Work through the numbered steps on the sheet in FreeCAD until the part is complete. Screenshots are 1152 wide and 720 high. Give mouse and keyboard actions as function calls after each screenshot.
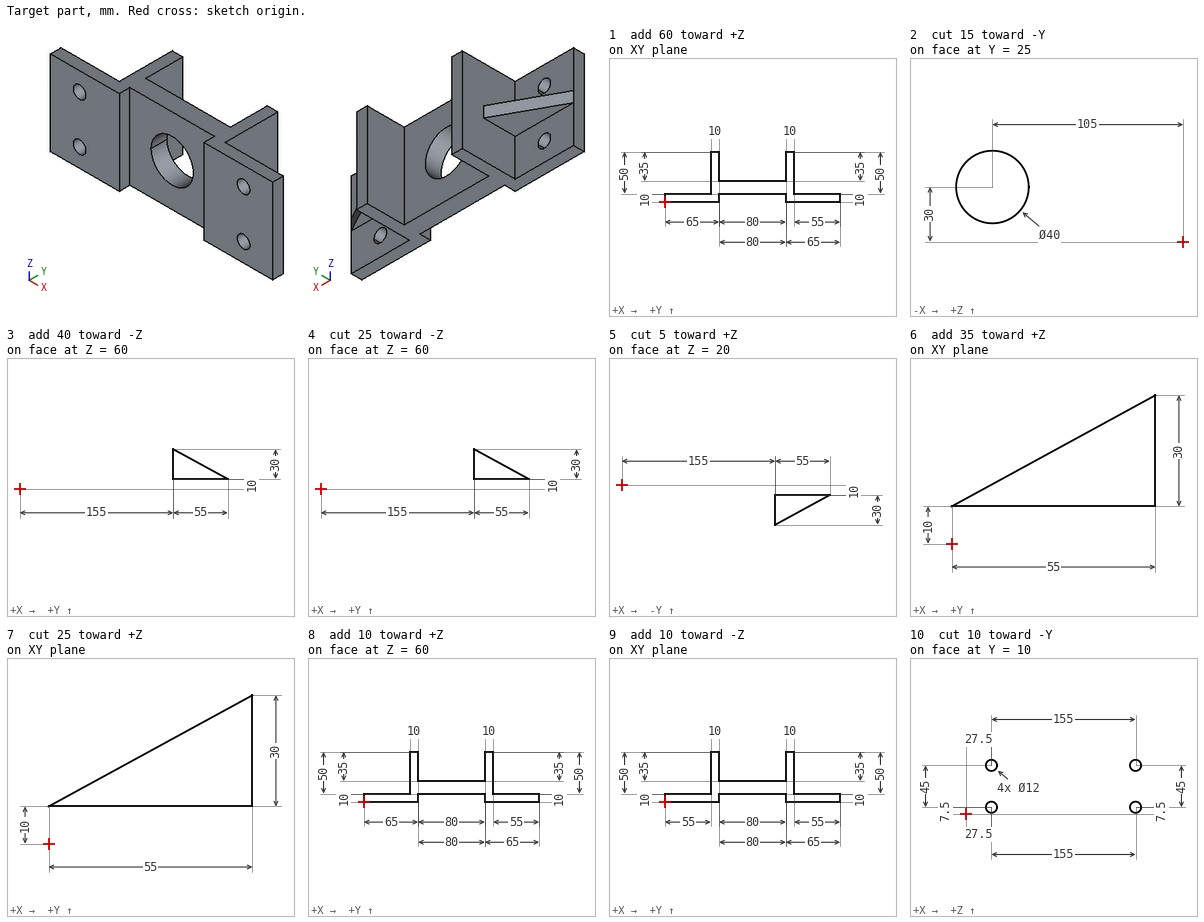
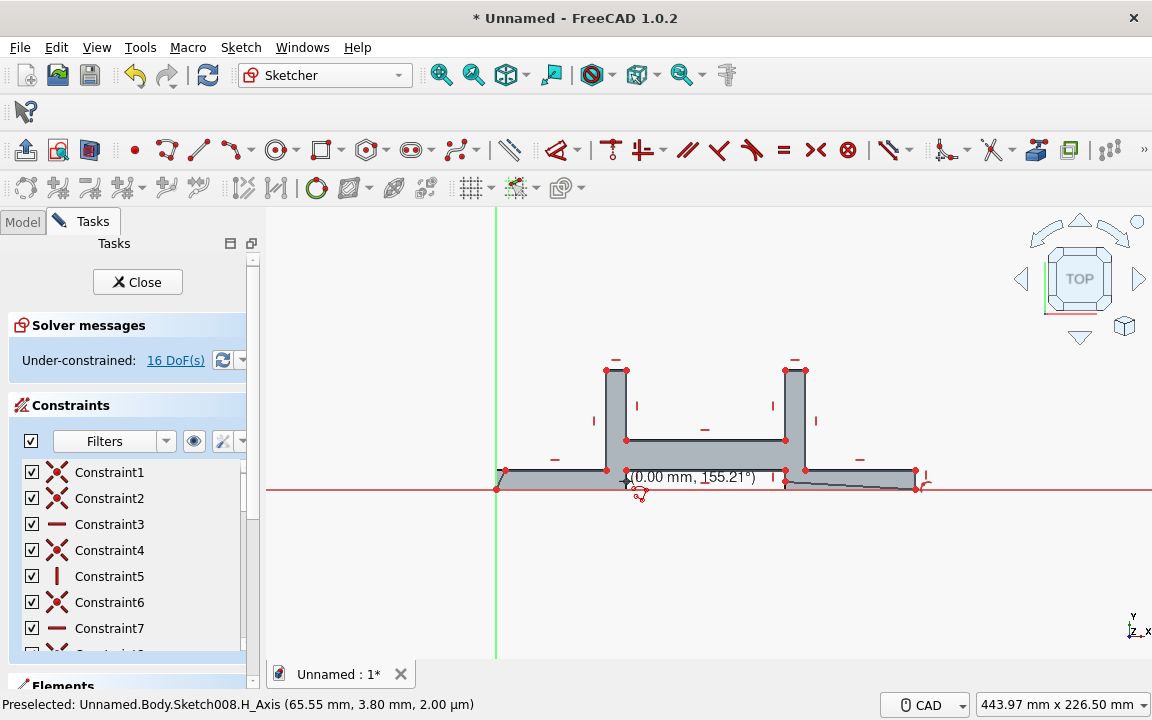
scroll(496, 490, up, 3)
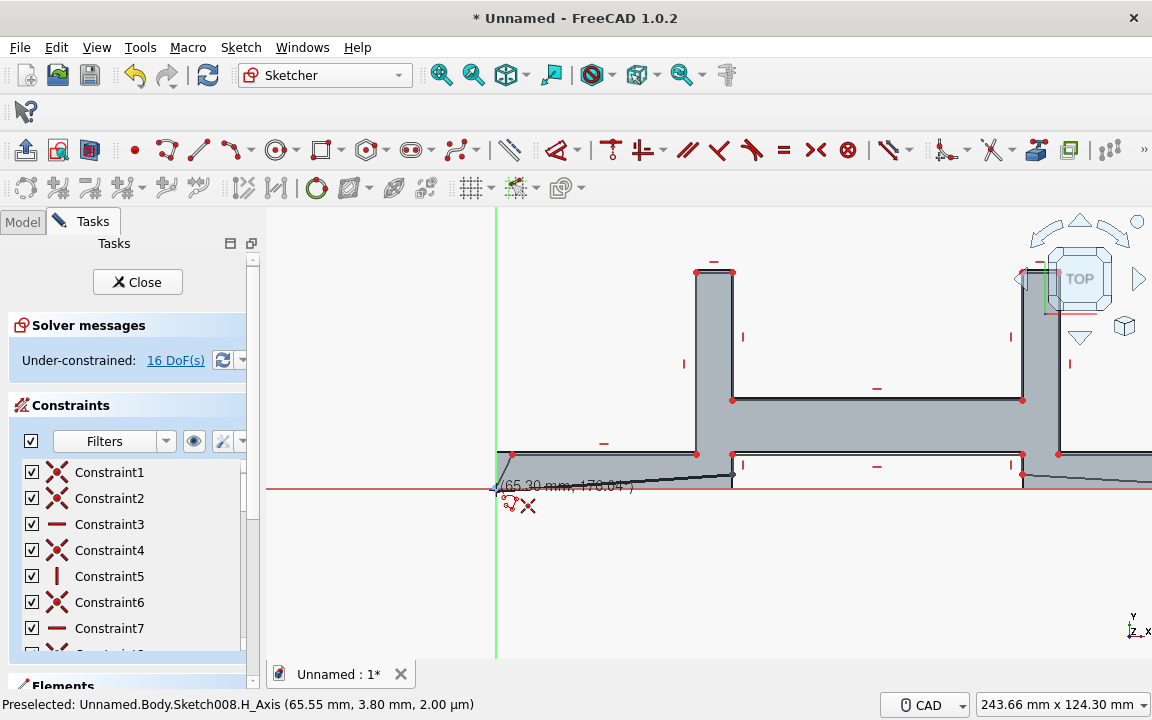
click(496, 489)
key(Escape)
key(Escape)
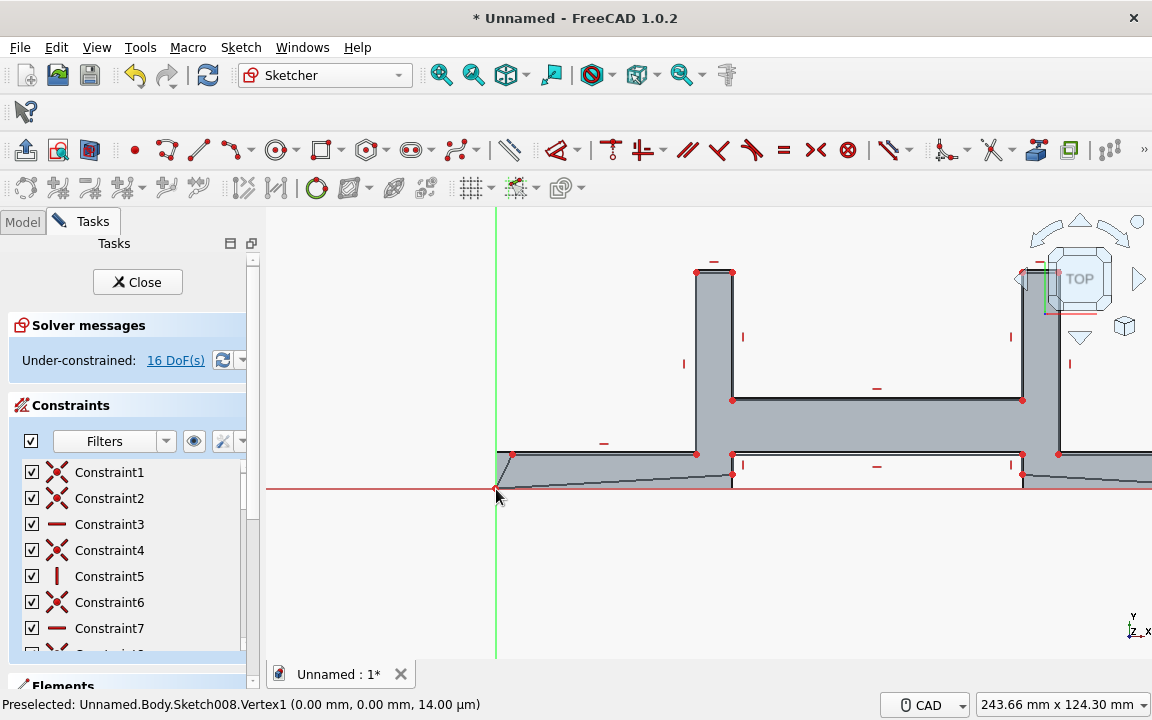
scroll(507, 465, up, 2)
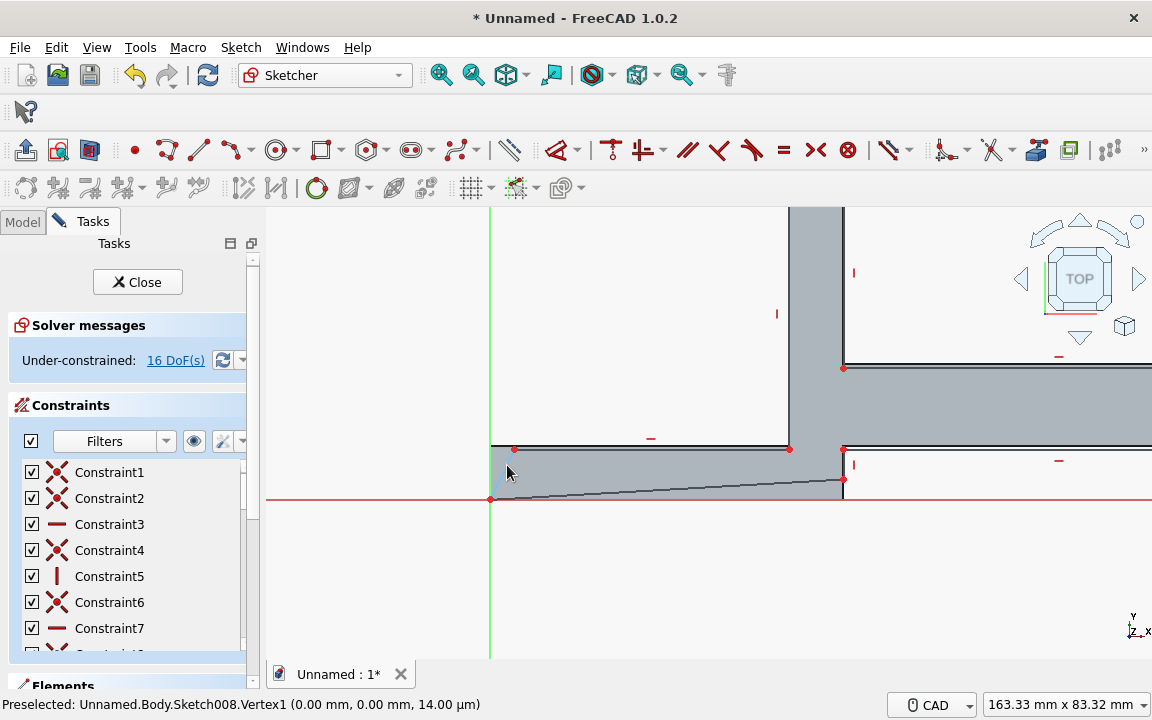
click(507, 465)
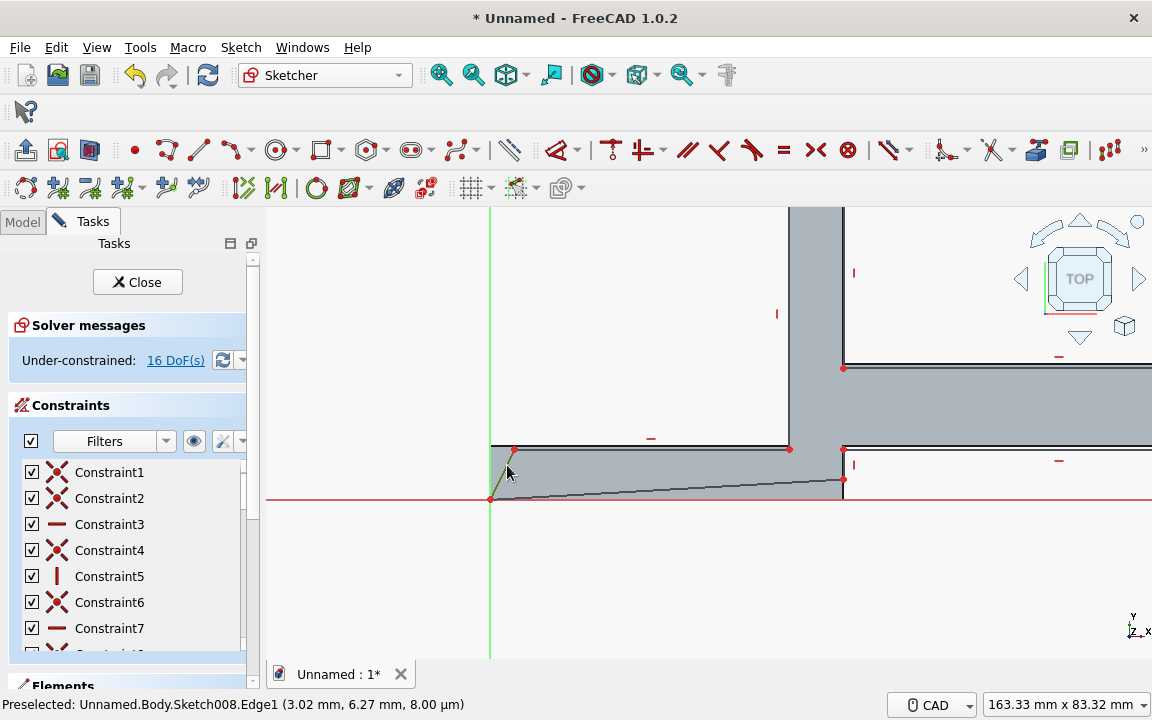
key(v)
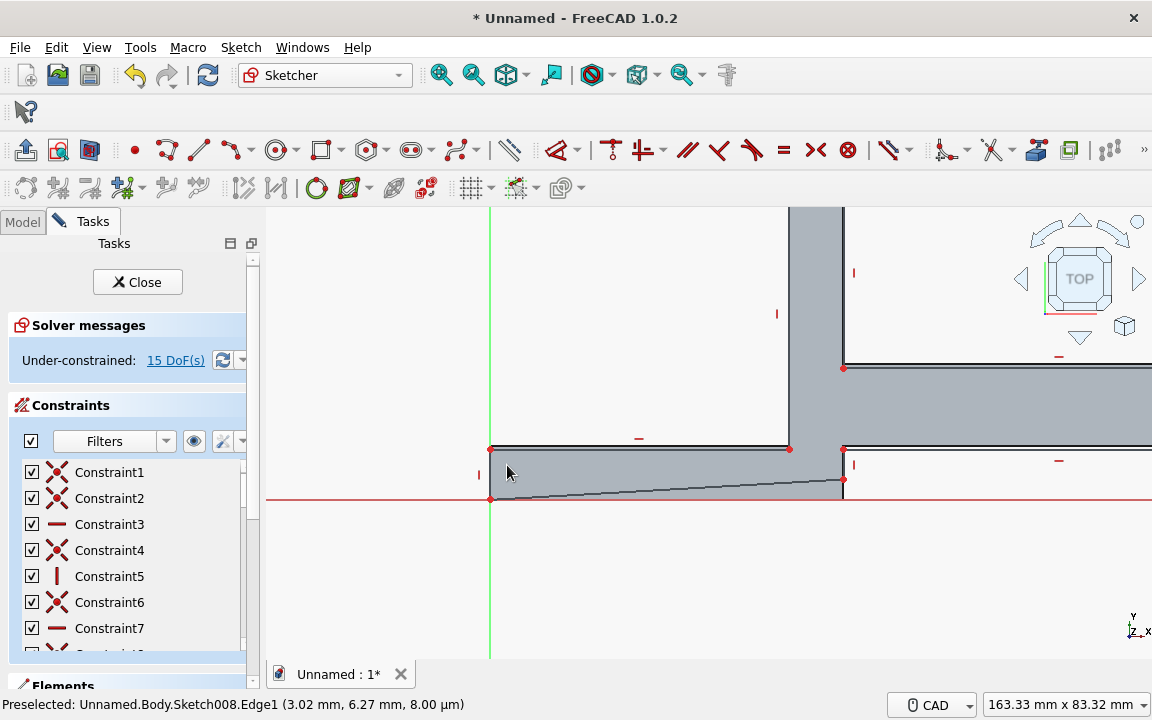
scroll(298, 511, down, 4)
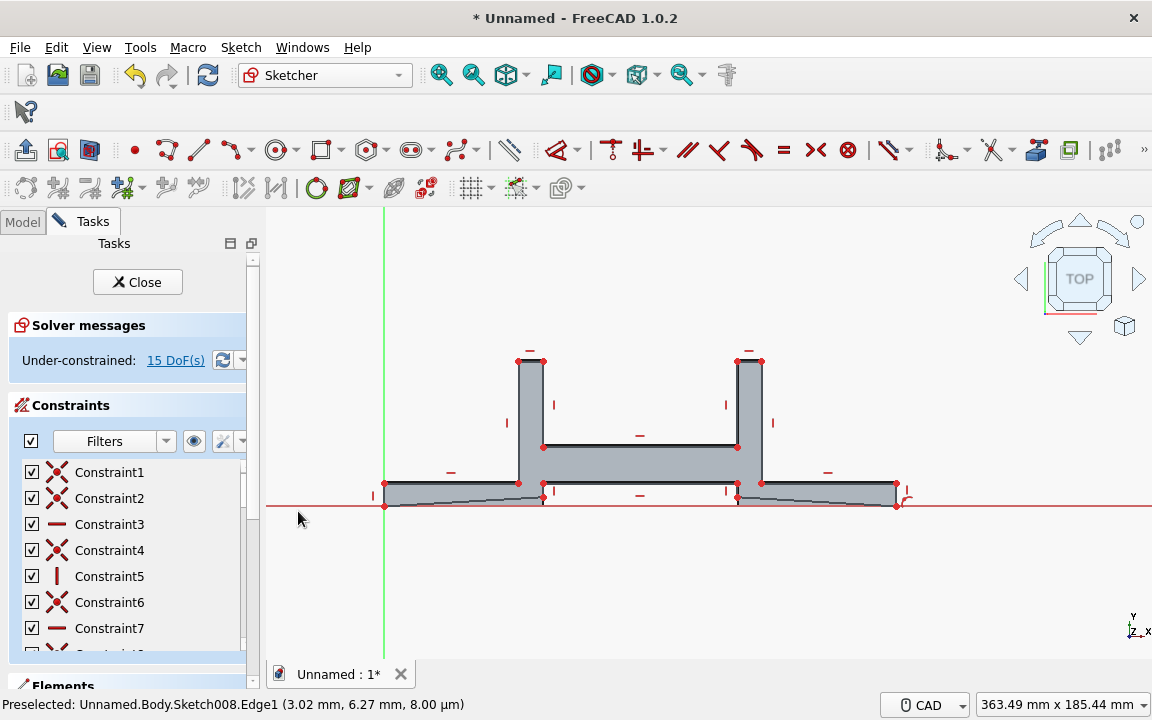
scroll(785, 500, up, 4)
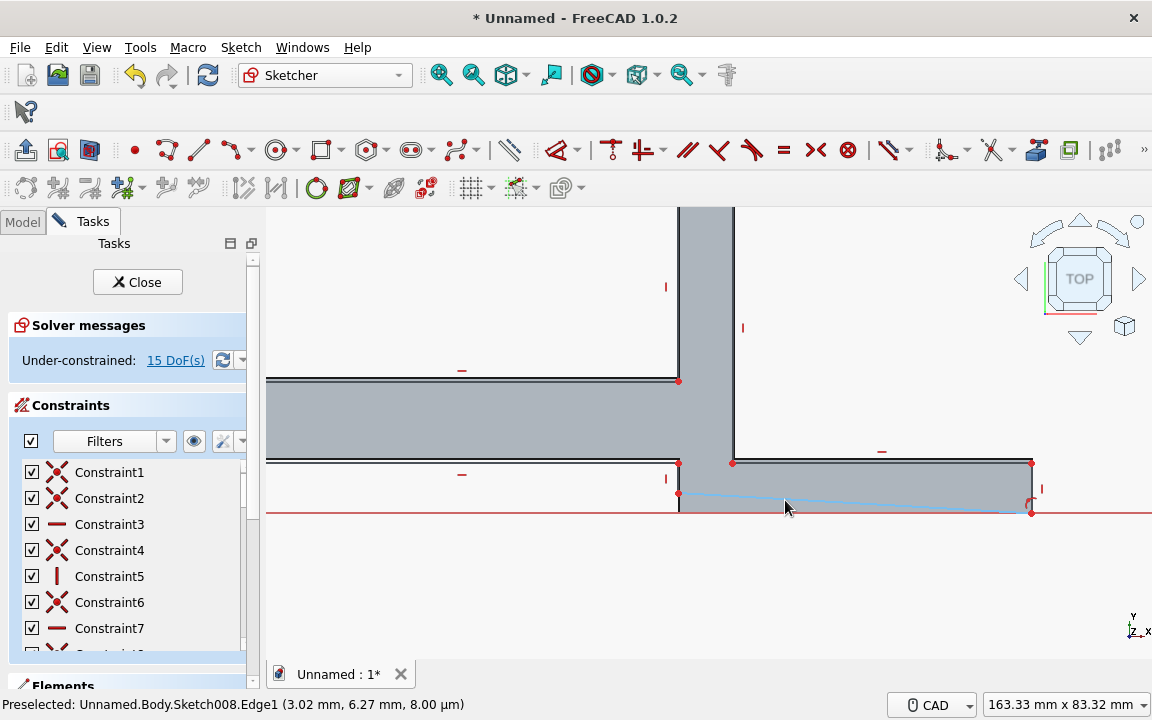
click(784, 499)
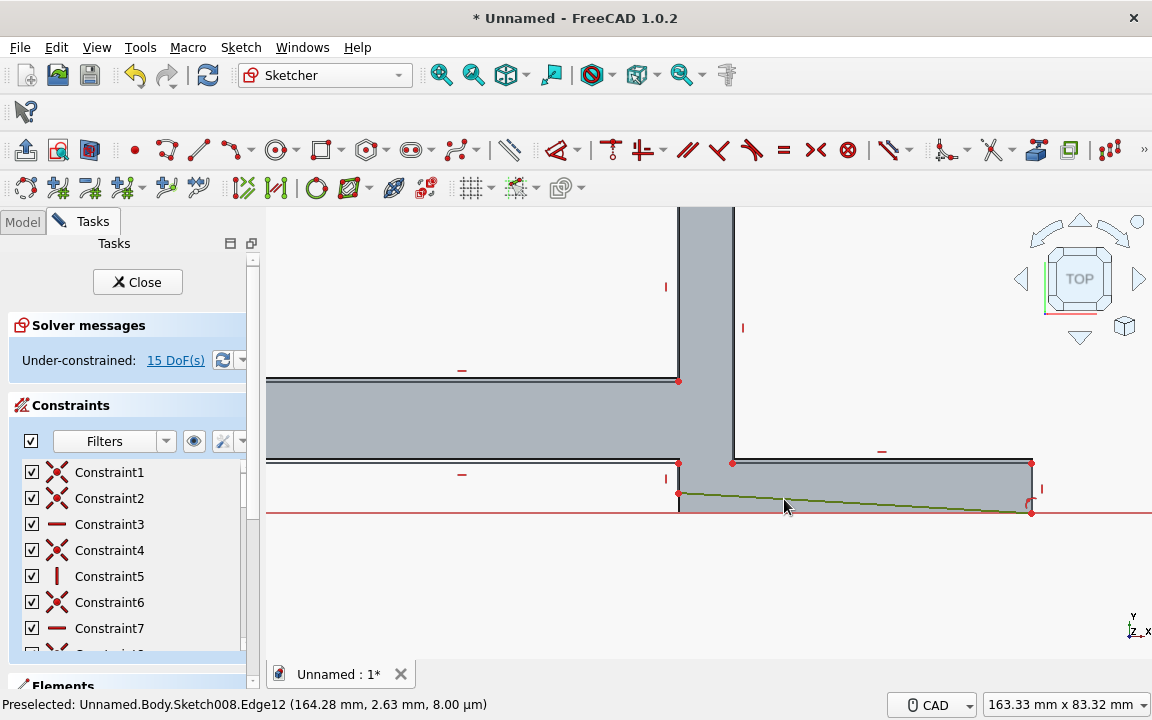
key(h)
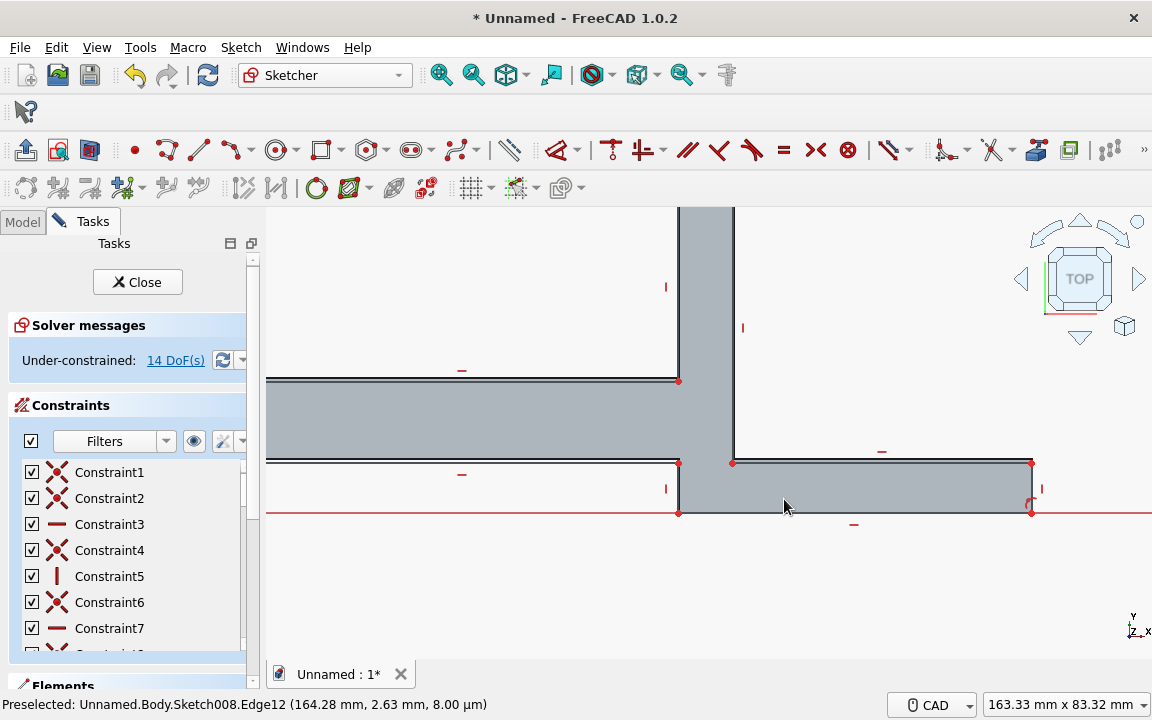
scroll(786, 500, down, 4)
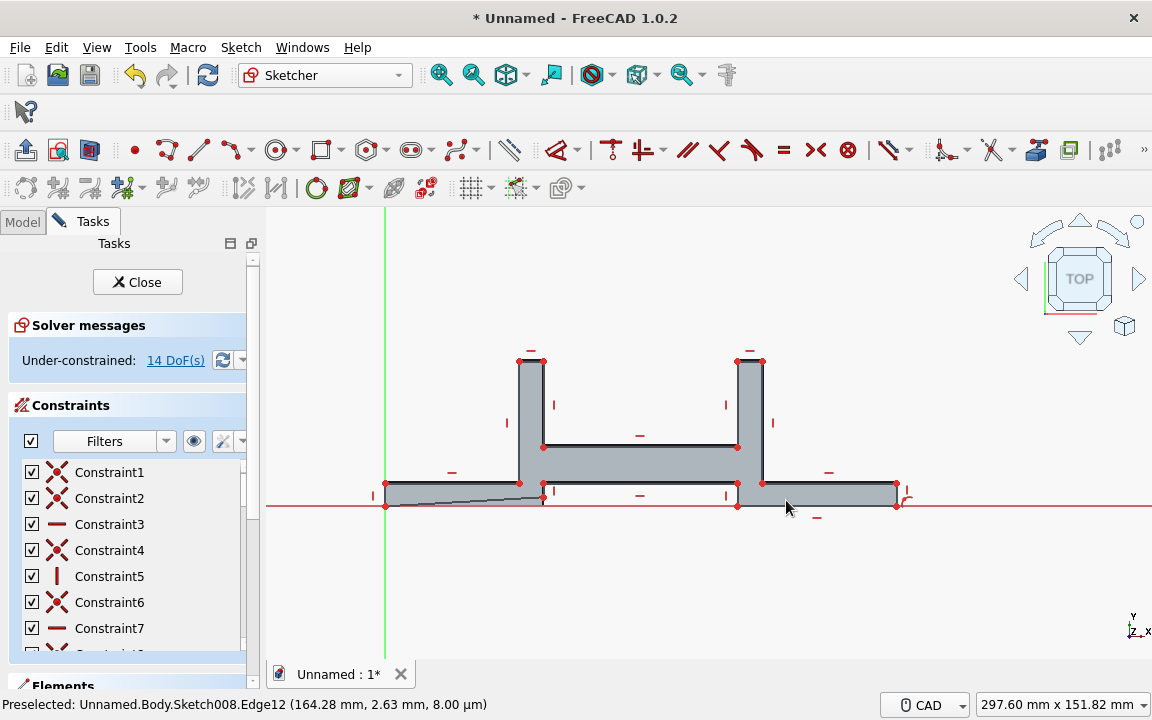
scroll(496, 500, up, 4)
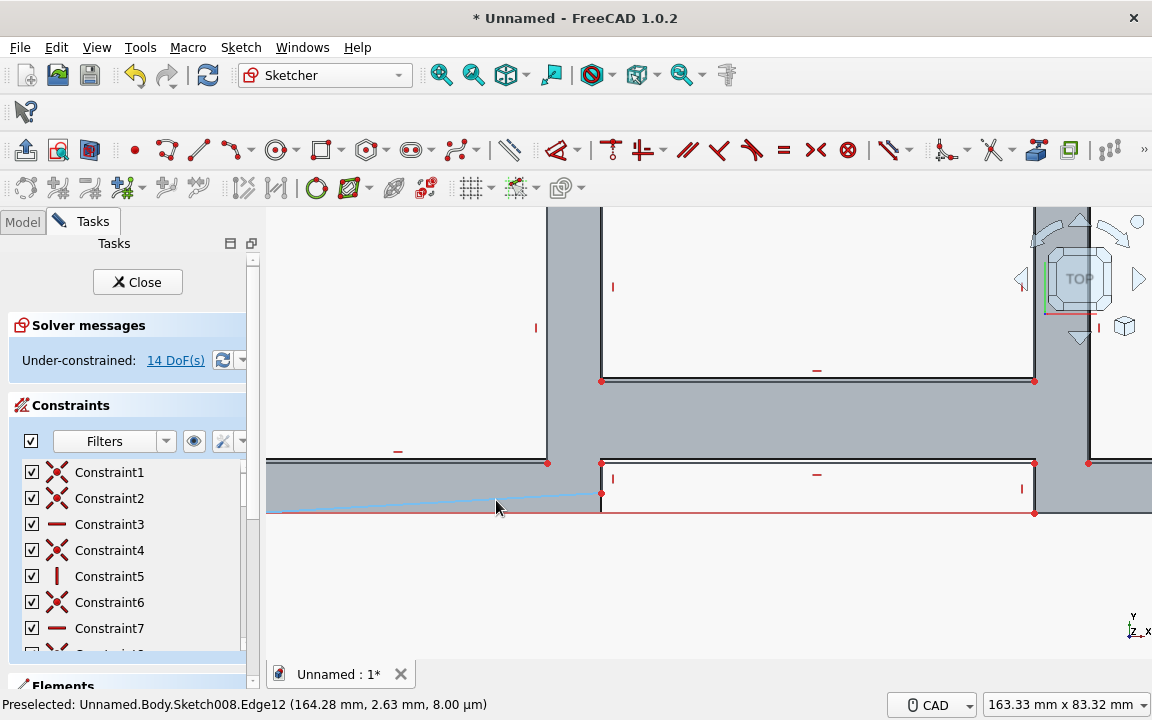
click(496, 499)